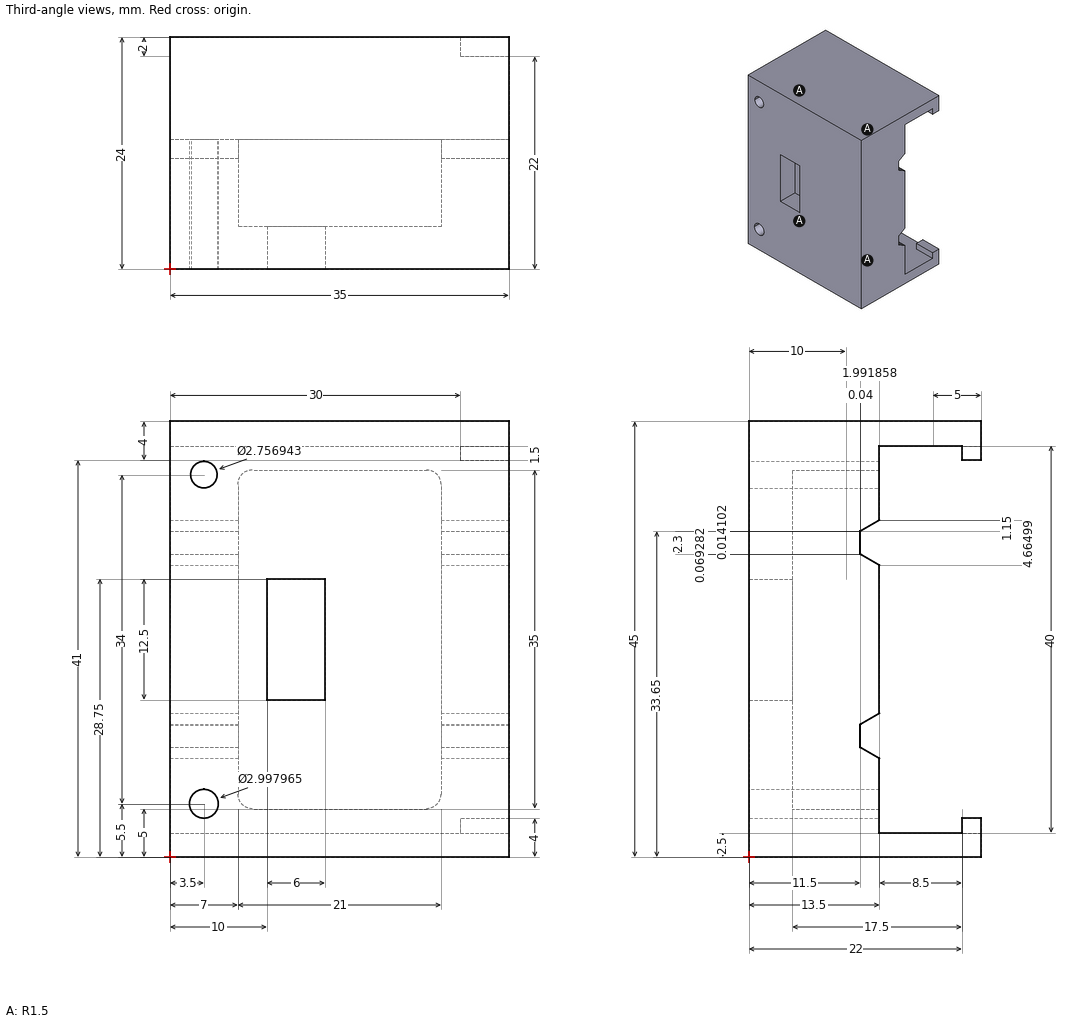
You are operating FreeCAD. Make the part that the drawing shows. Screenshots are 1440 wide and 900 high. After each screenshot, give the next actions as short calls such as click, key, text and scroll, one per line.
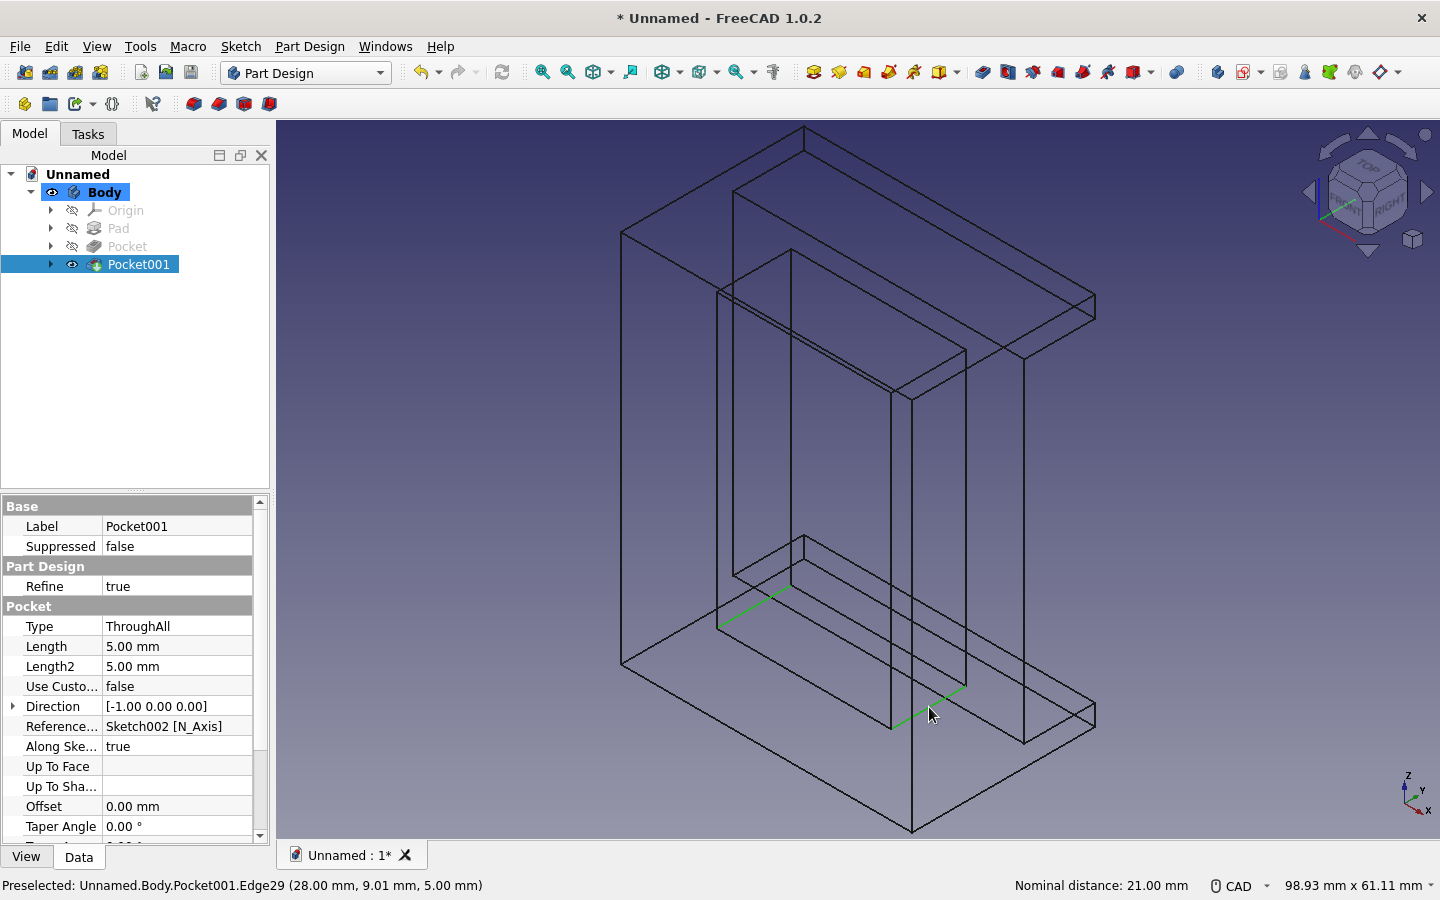
click(929, 370, ctrl)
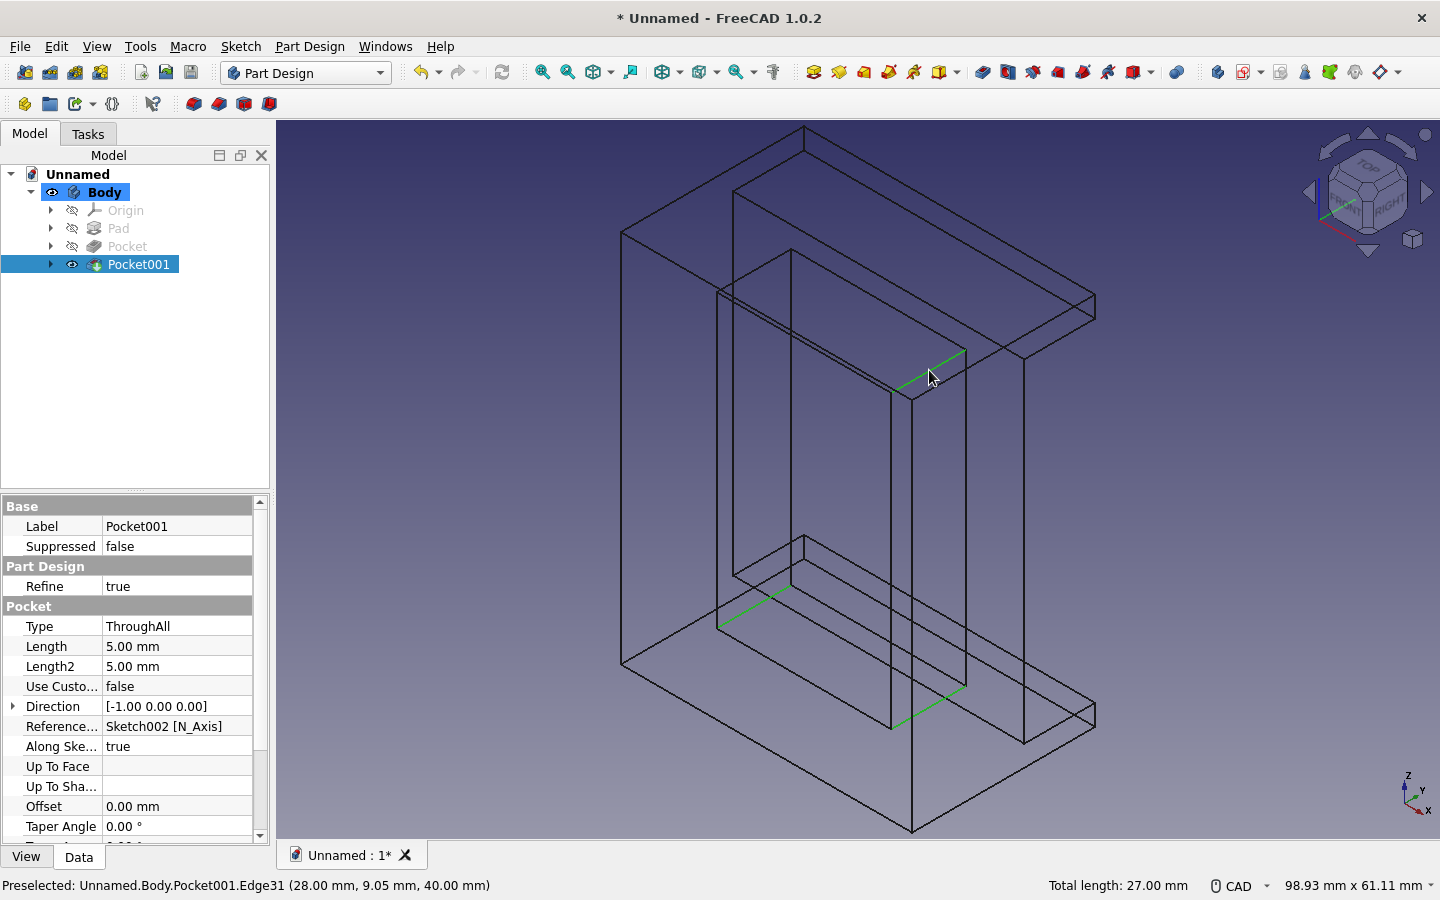
click(754, 270, ctrl)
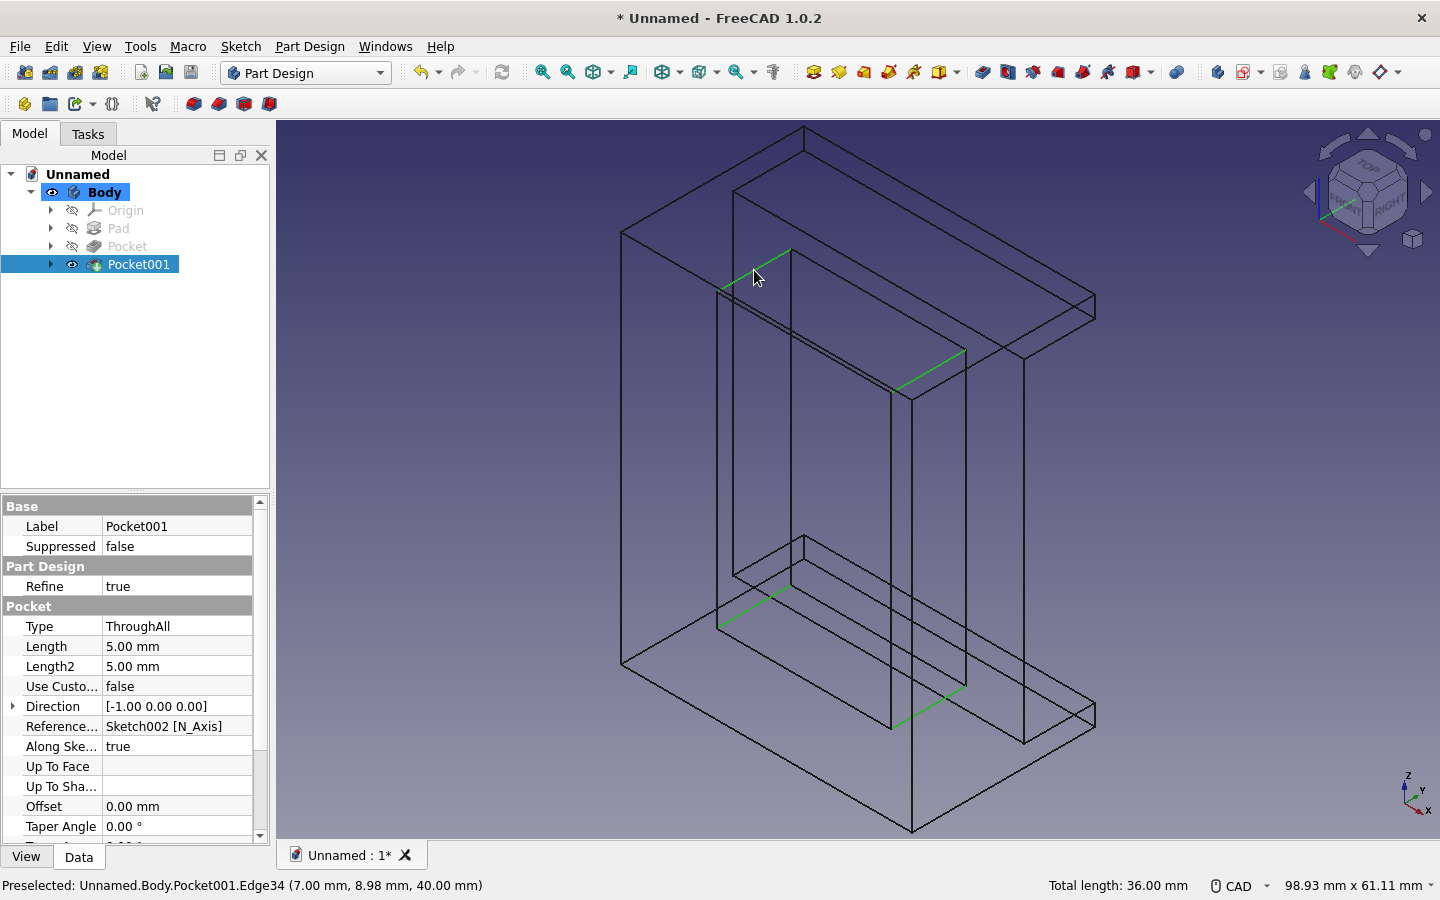
key(v)
key(1)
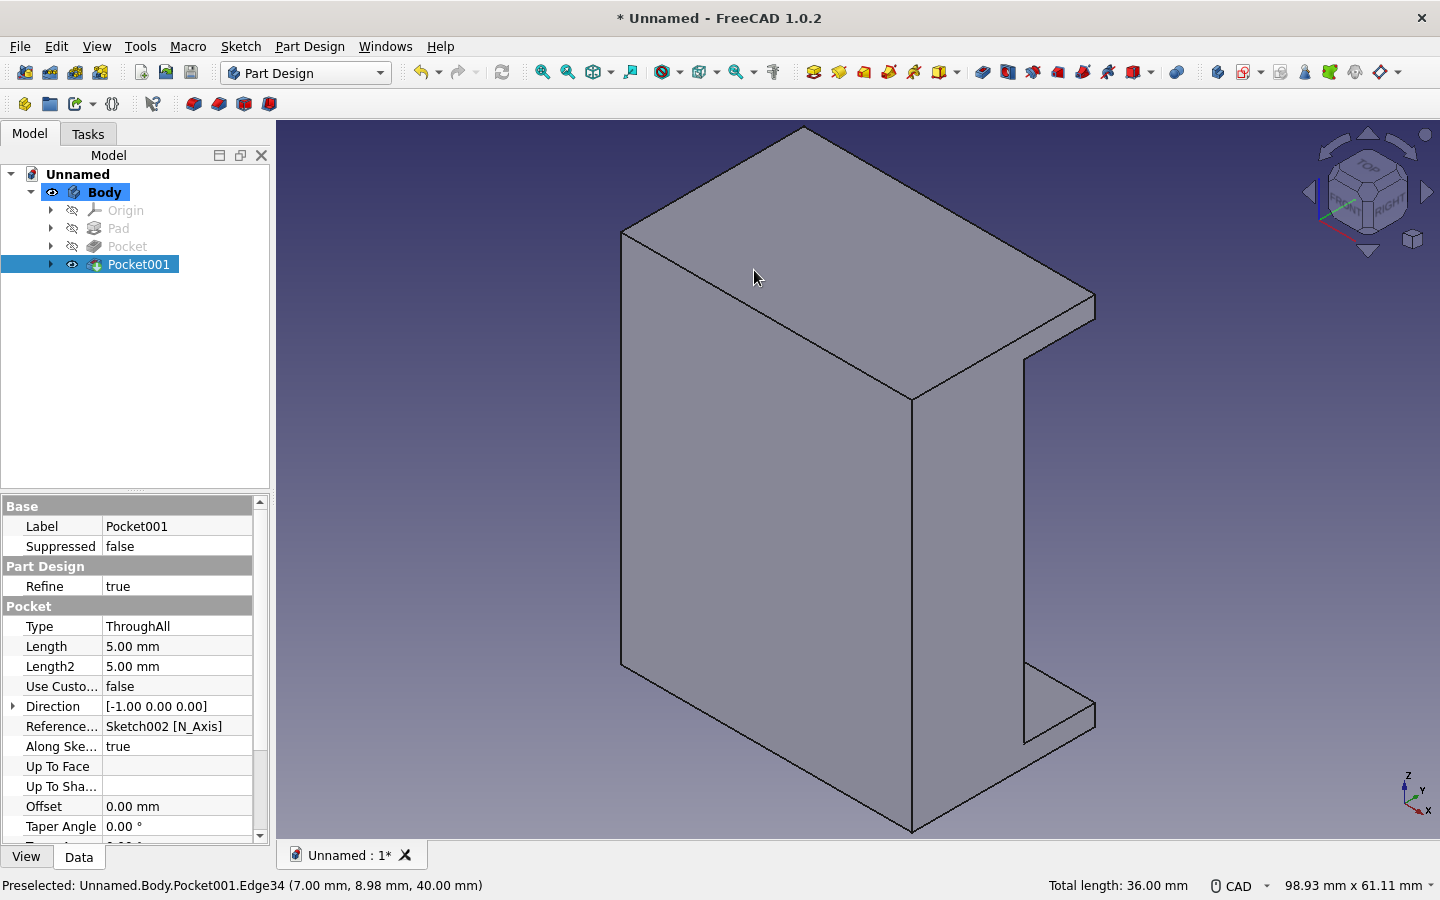
click(194, 104)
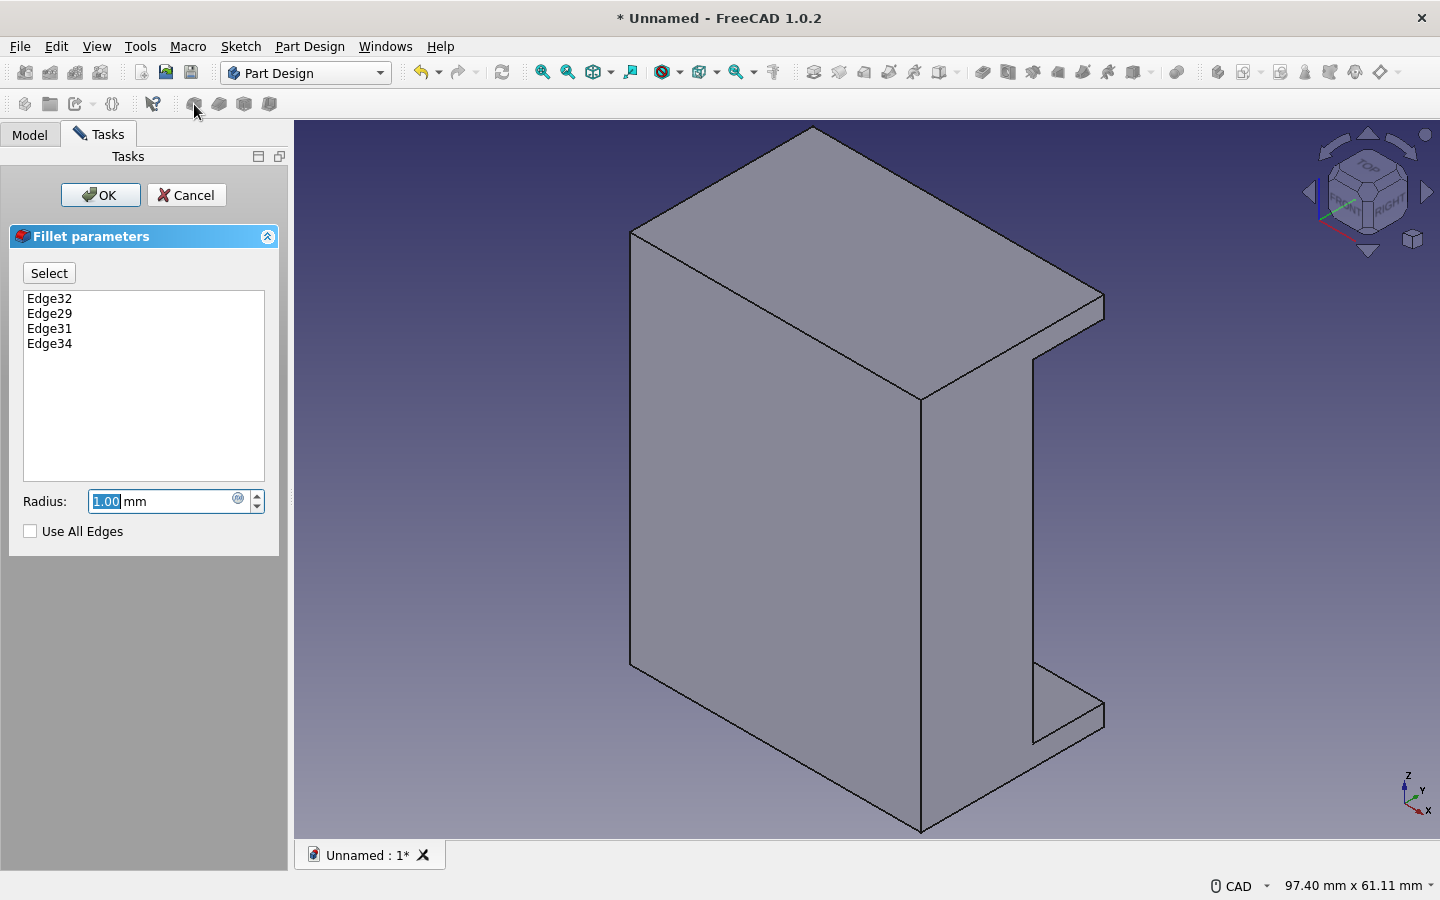
text(1.5)
key(Tab)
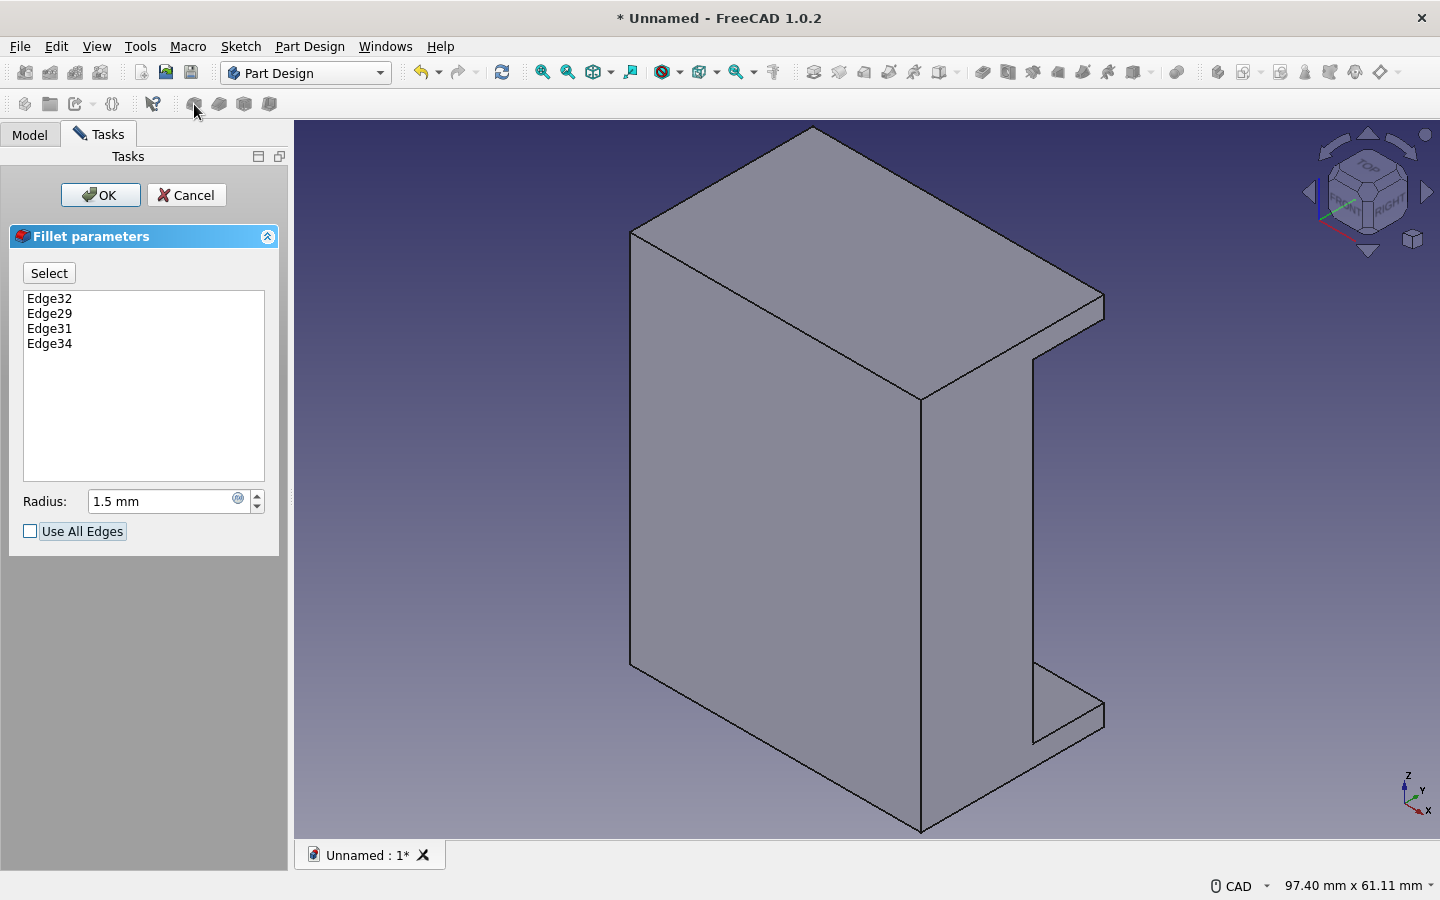
click(101, 195)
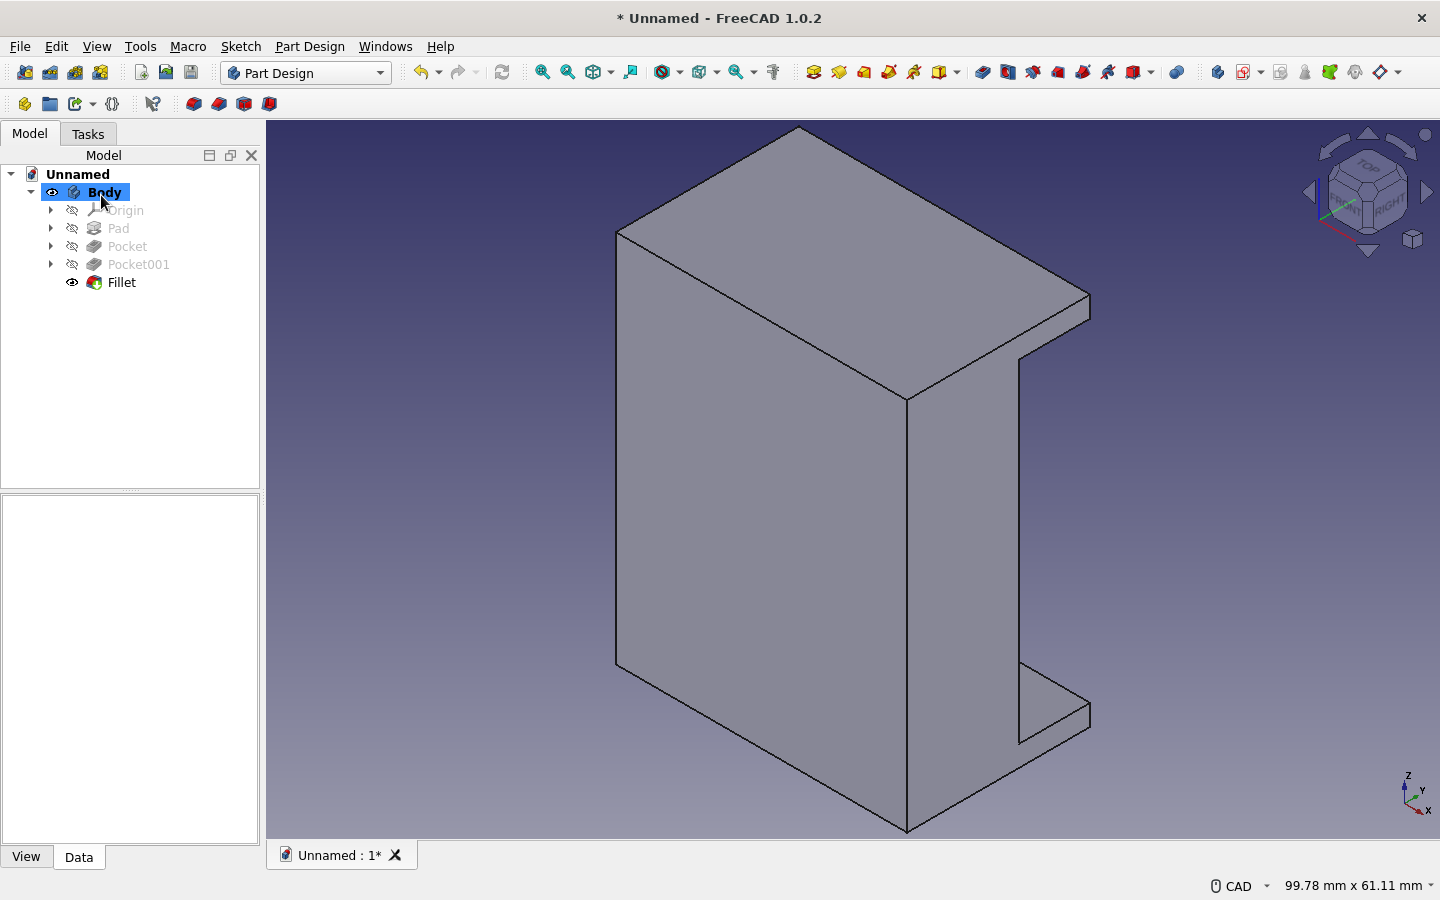
click(895, 286)